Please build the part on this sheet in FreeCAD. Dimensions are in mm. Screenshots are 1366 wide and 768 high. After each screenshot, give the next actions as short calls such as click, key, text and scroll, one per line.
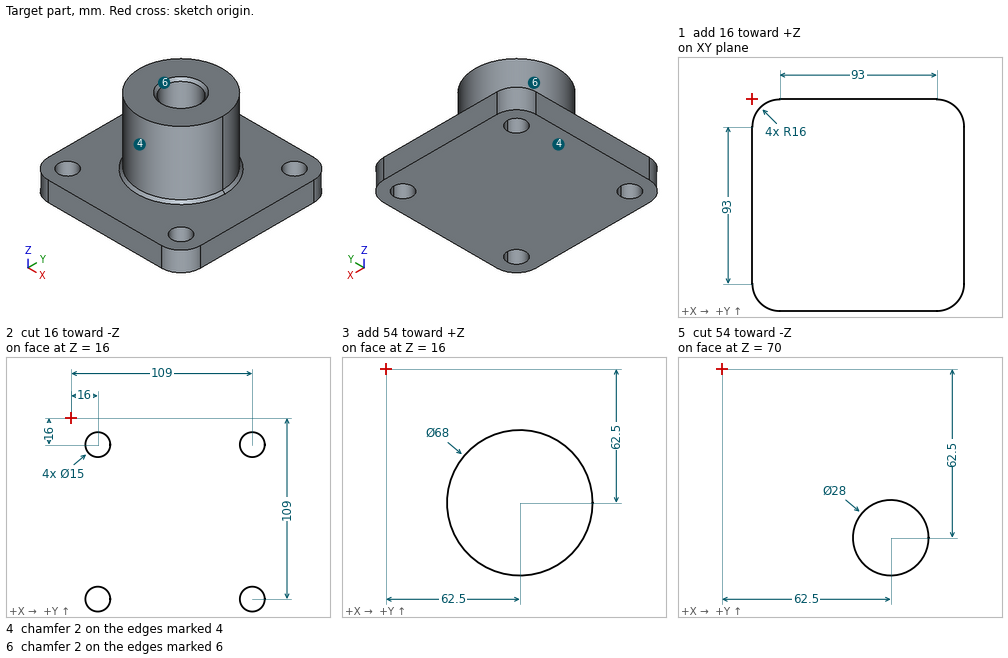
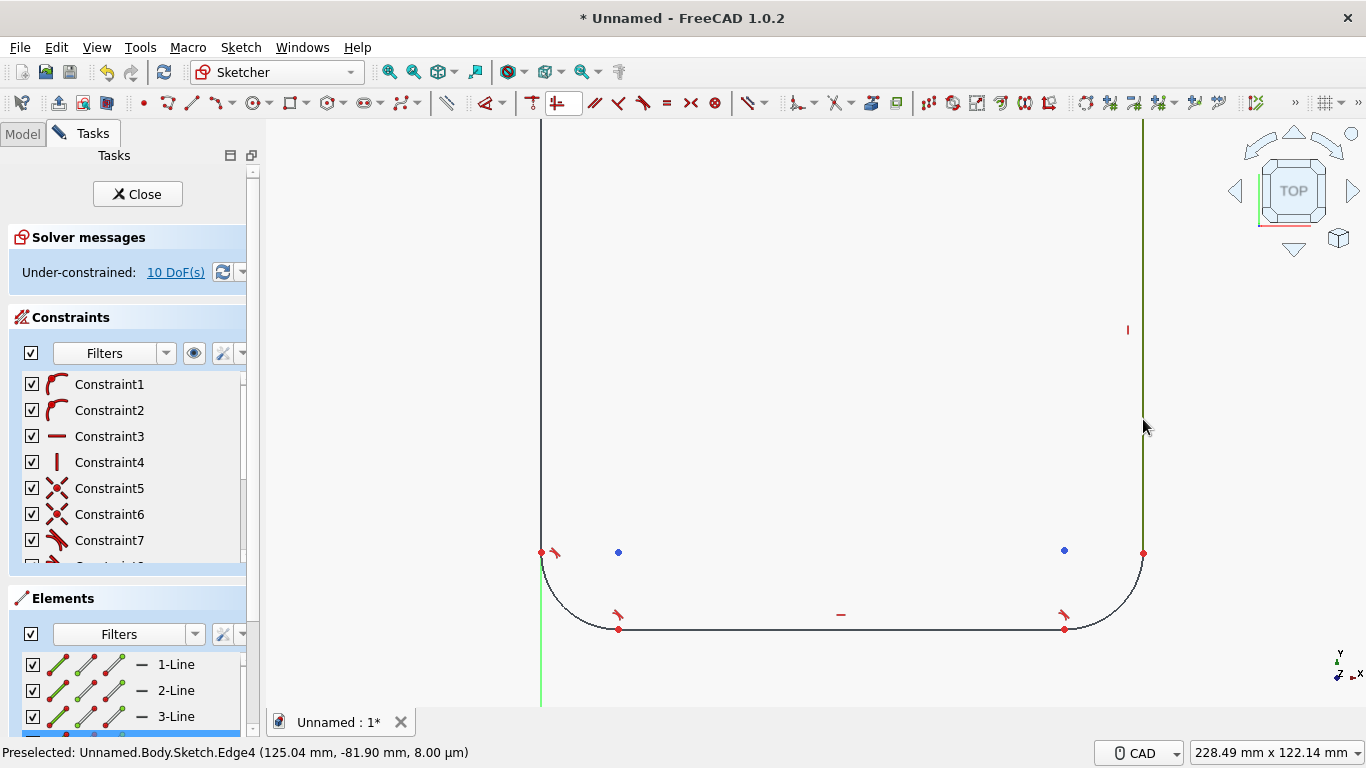
click(1099, 621)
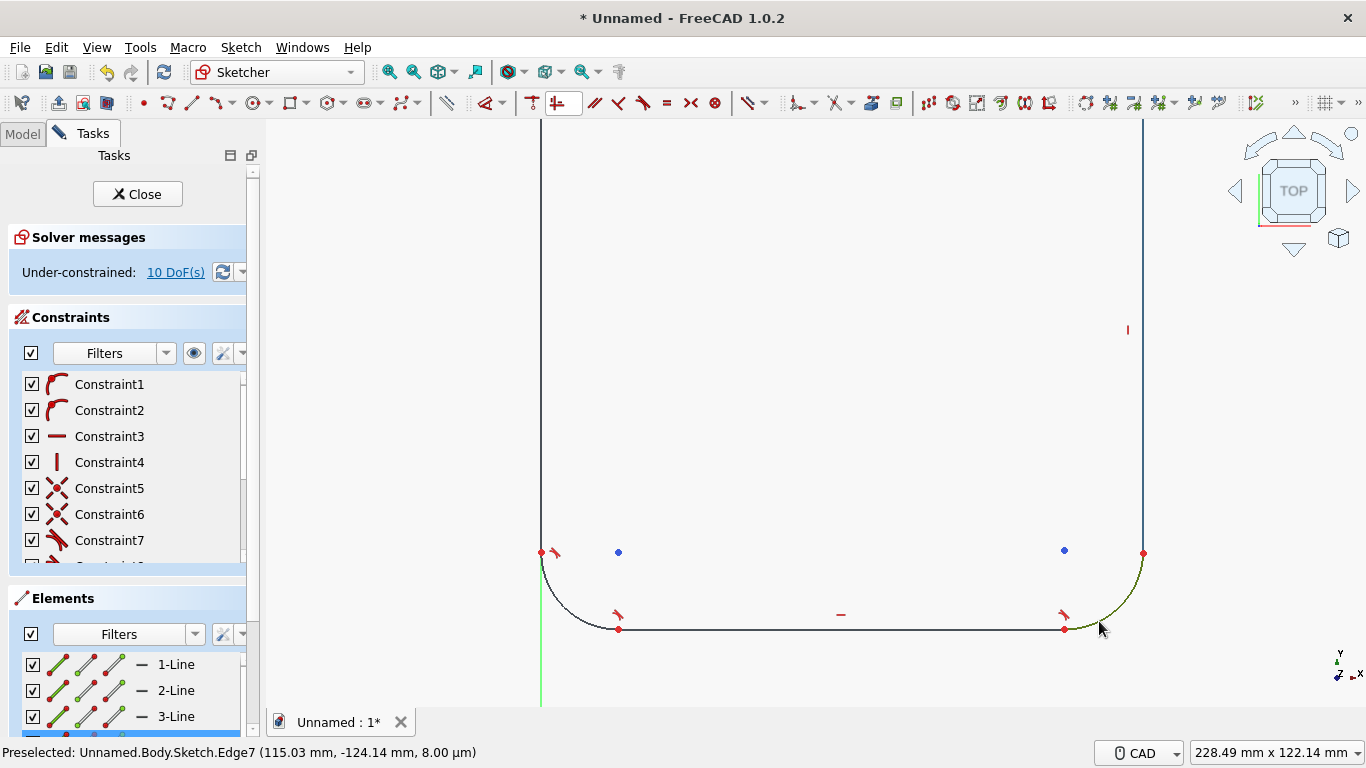
click(644, 104)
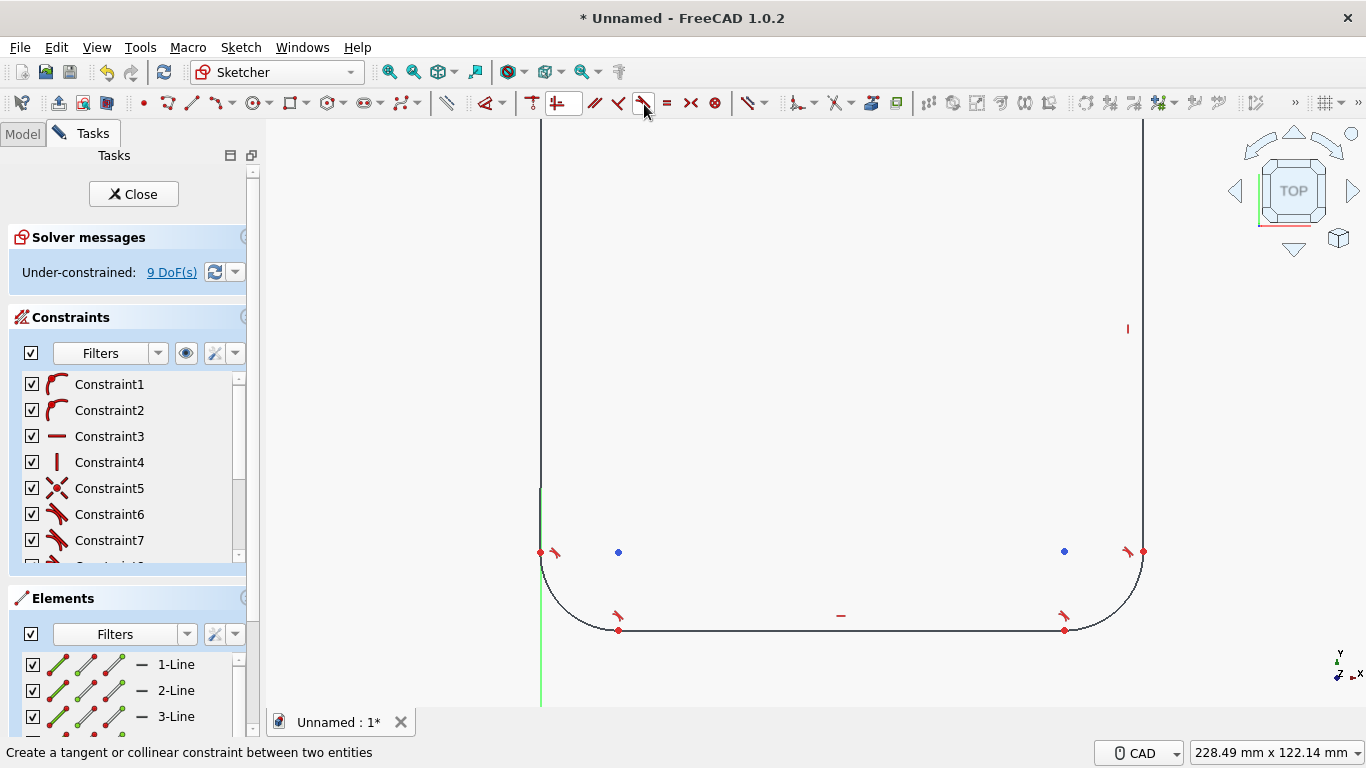
click(1143, 418)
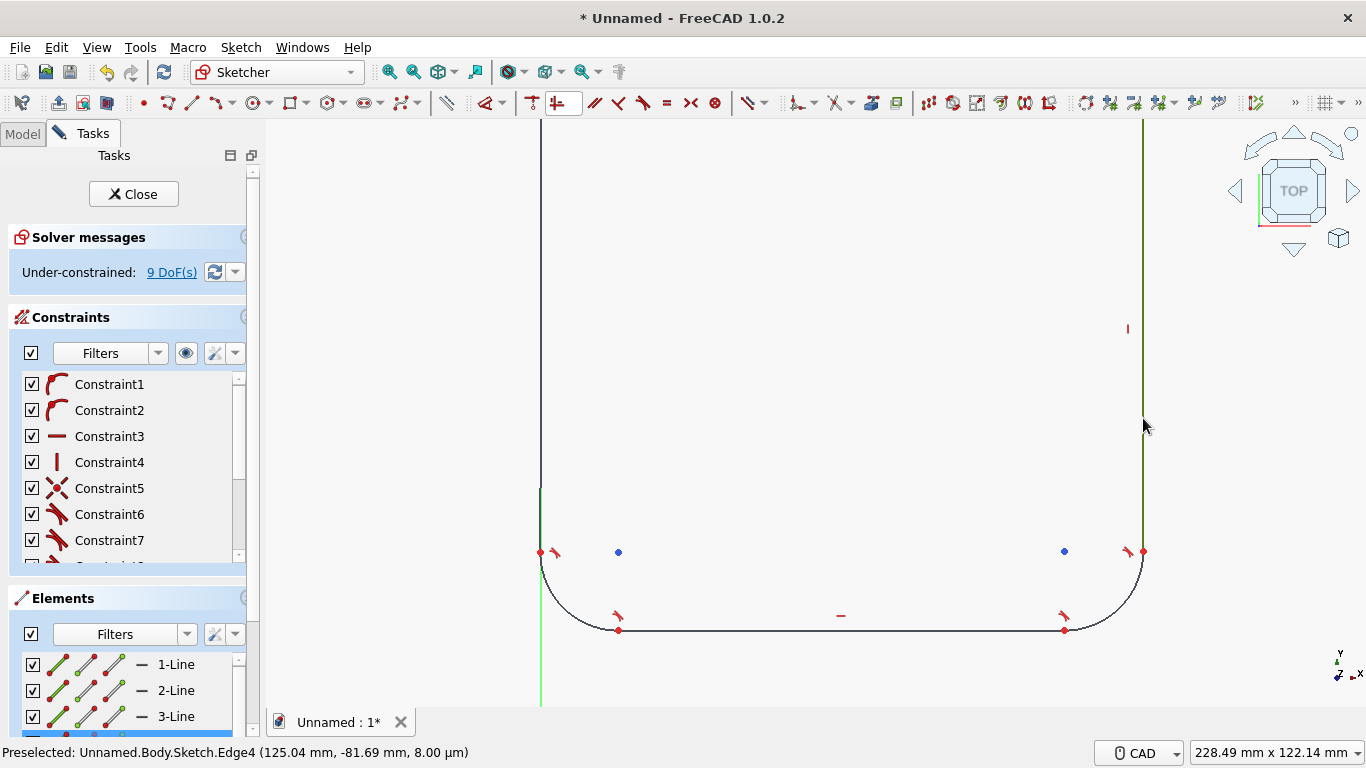
scroll(555, 589, down, 2)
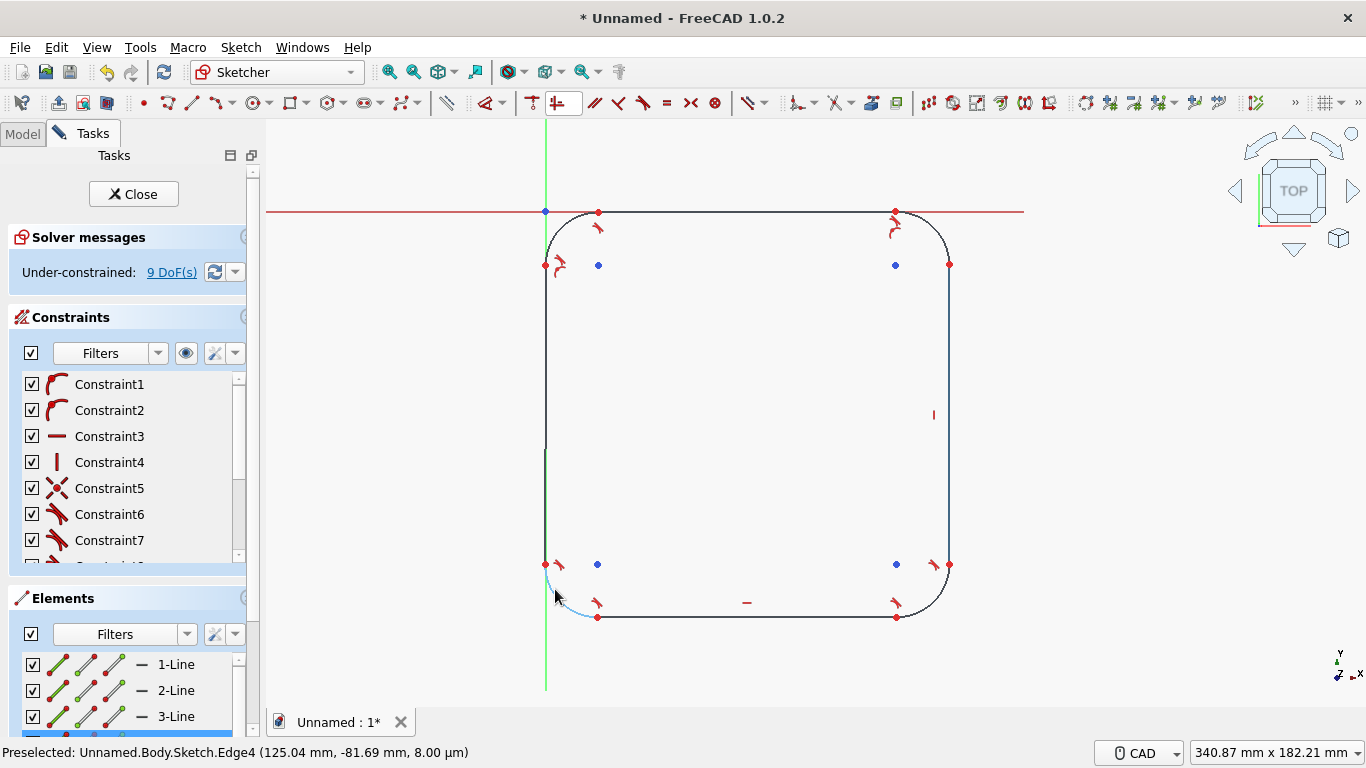
click(943, 241)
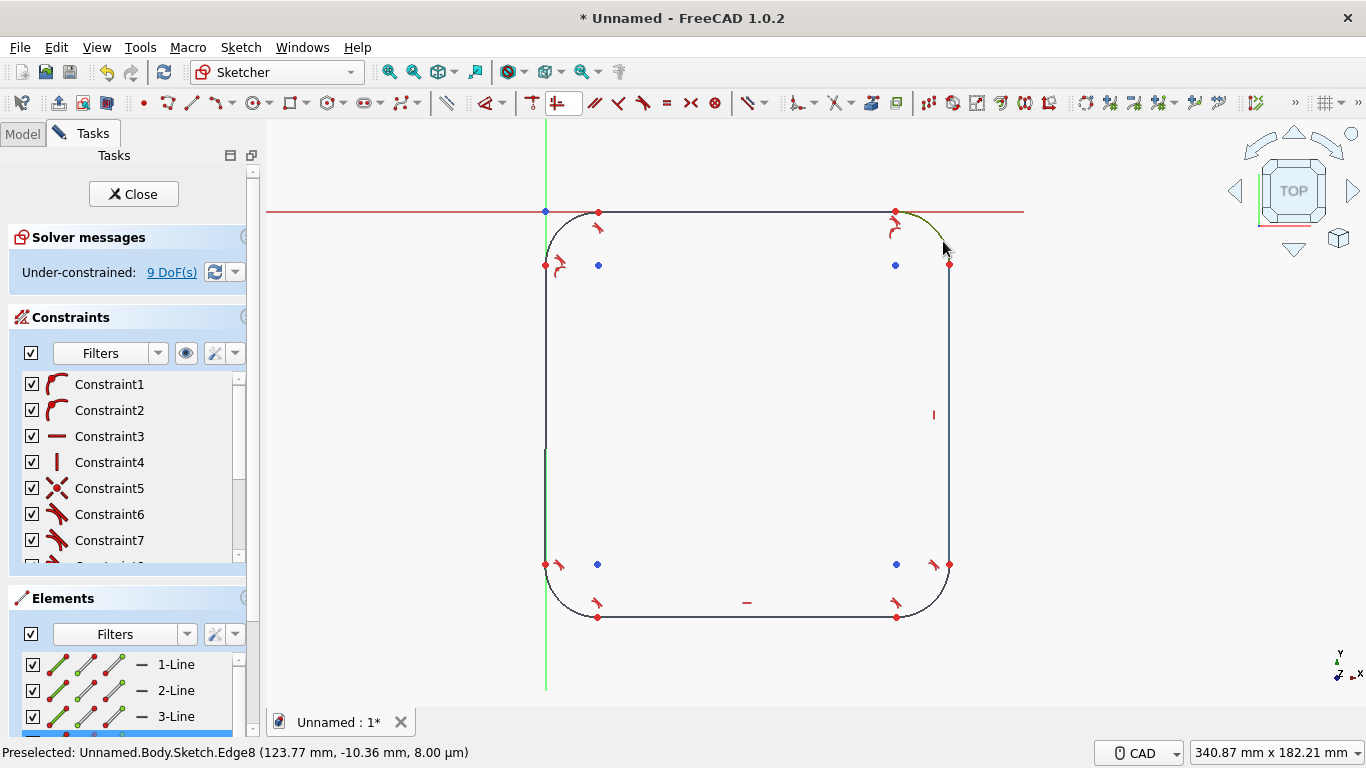
key(t)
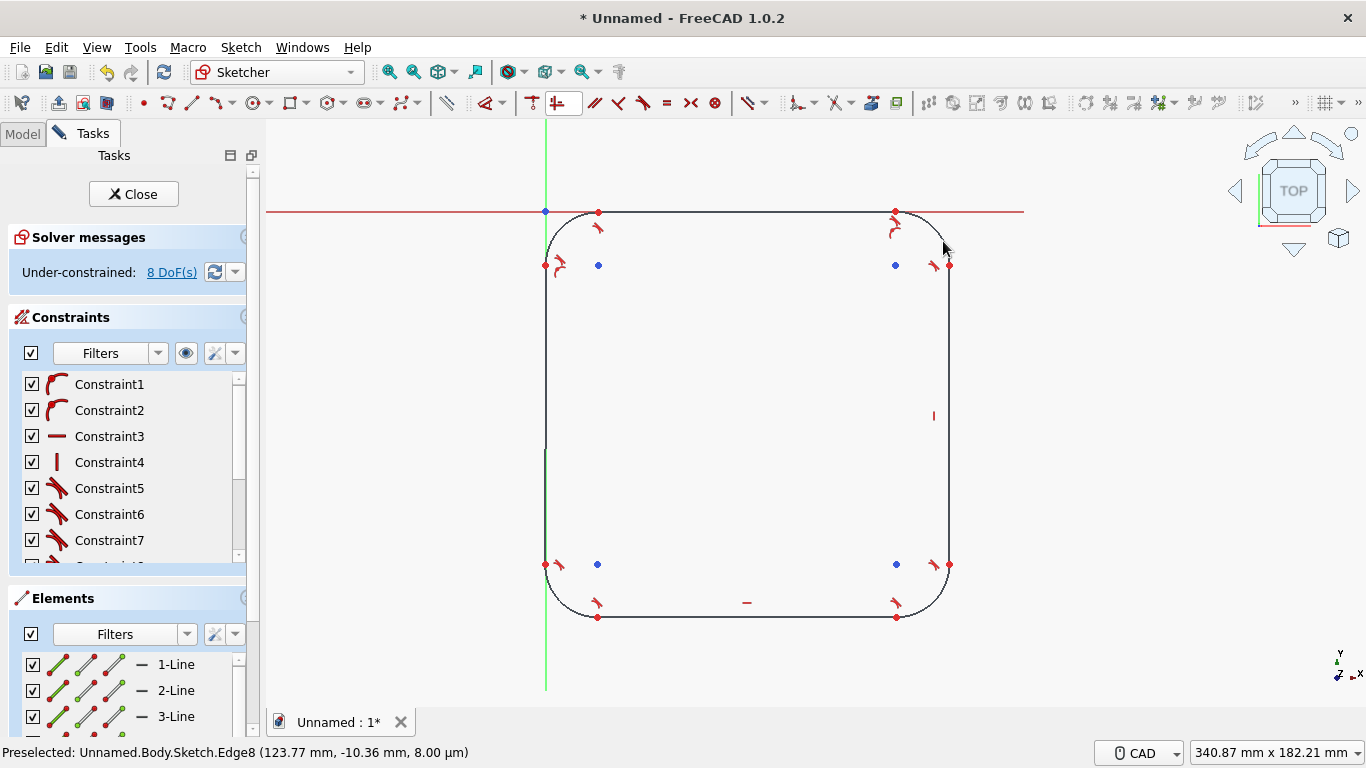
click(806, 212)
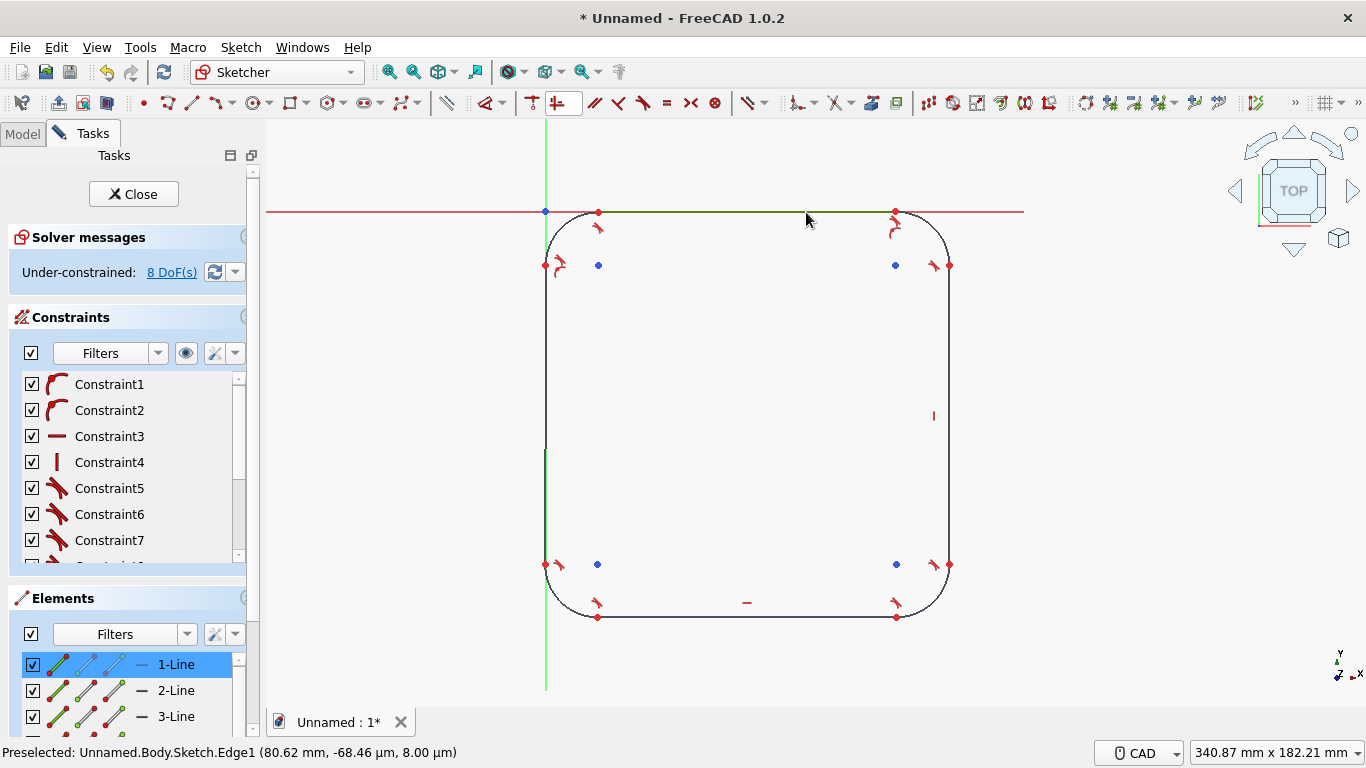
key(h)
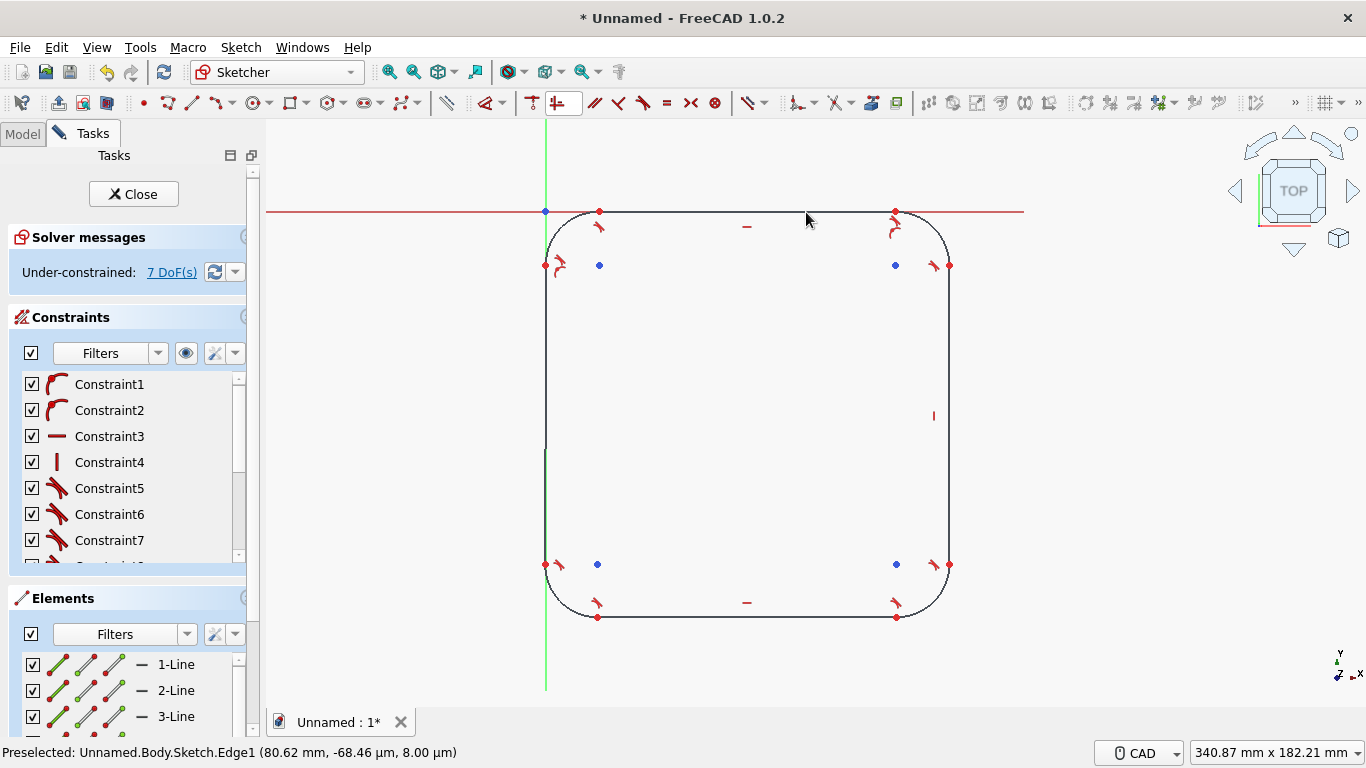
click(546, 355)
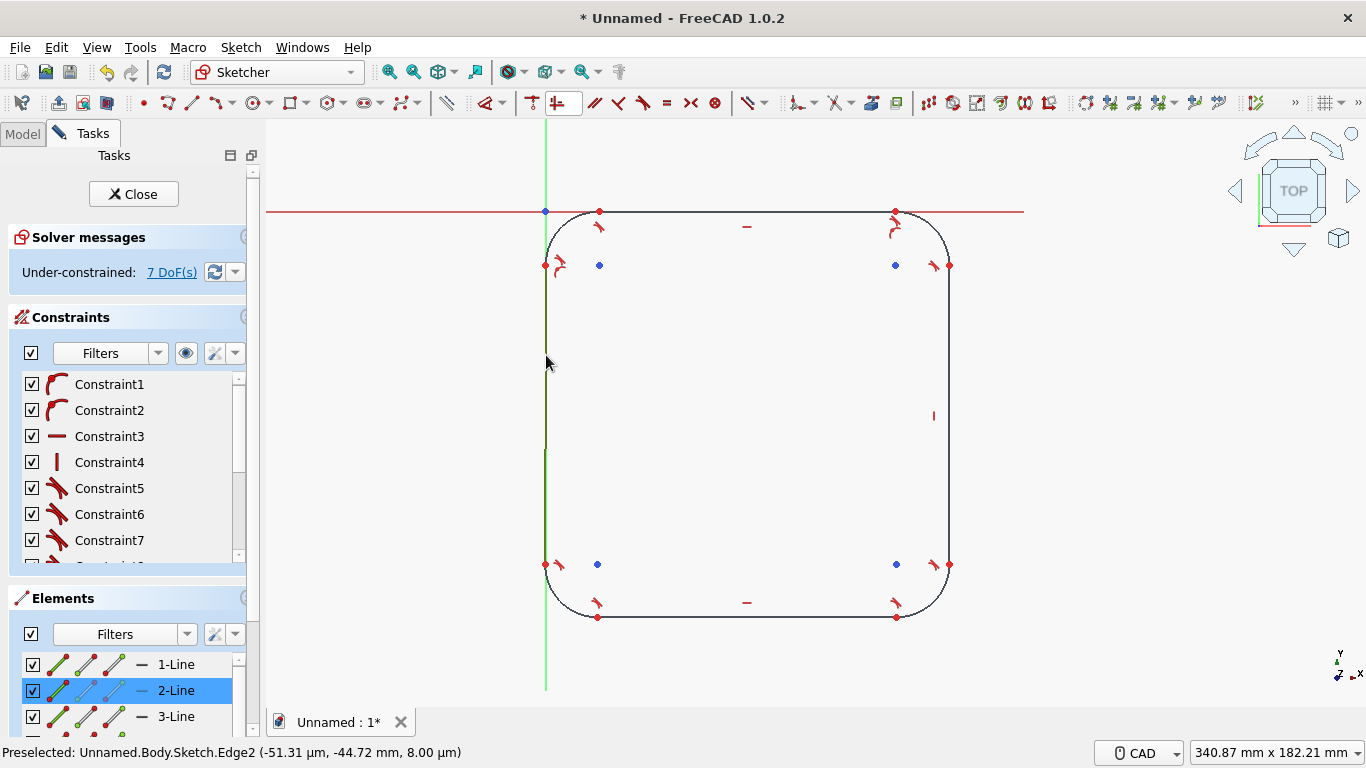
click(576, 104)